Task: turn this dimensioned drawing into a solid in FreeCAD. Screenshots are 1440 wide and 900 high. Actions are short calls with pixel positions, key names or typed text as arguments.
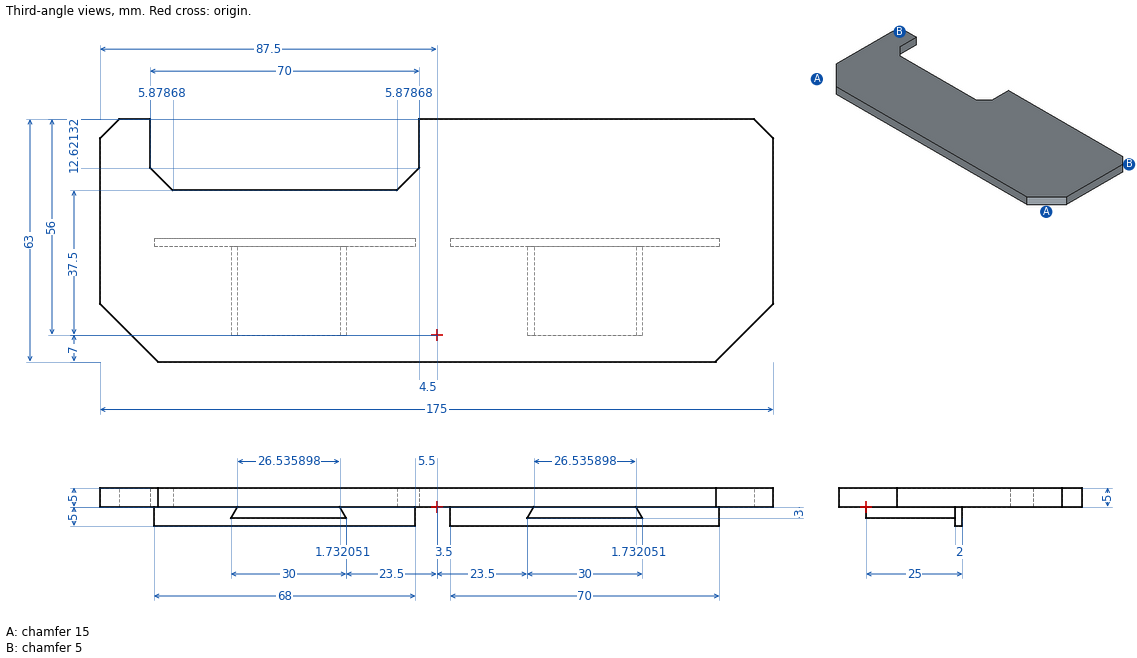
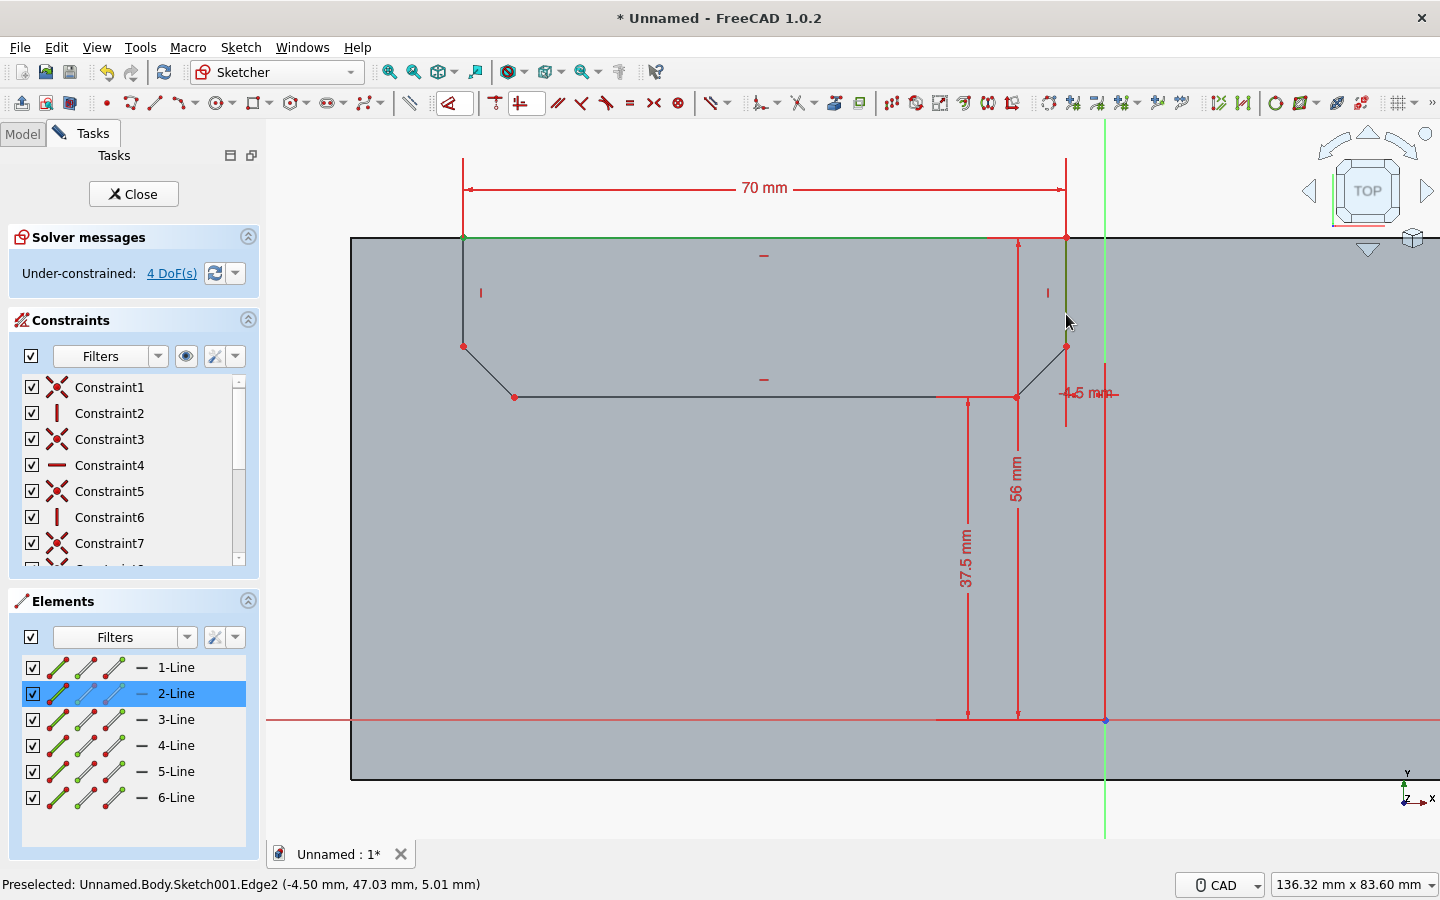
key(i)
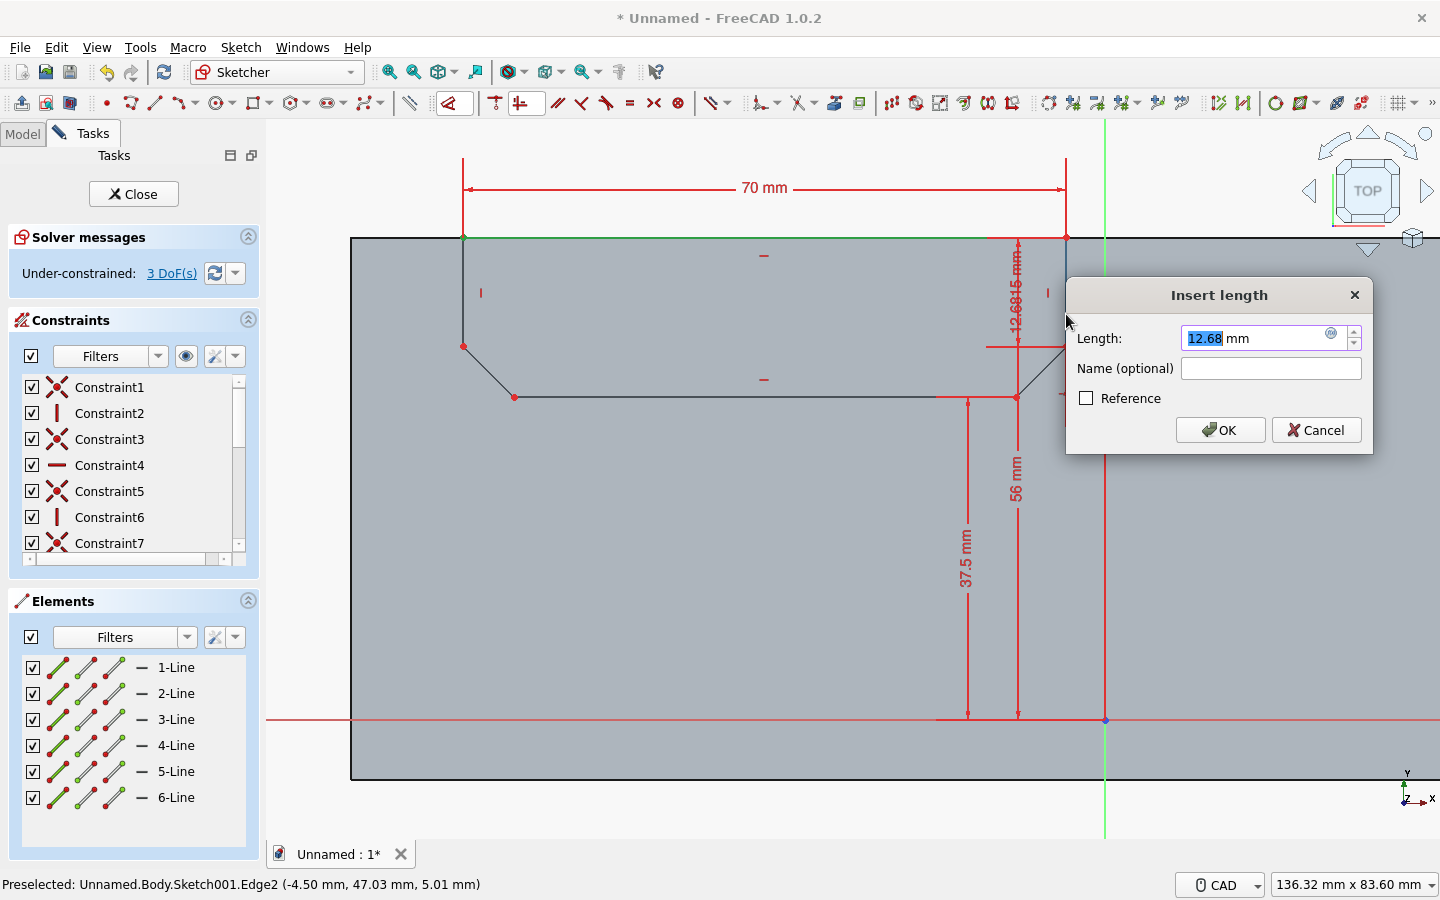
text(12.62132)
key(Return)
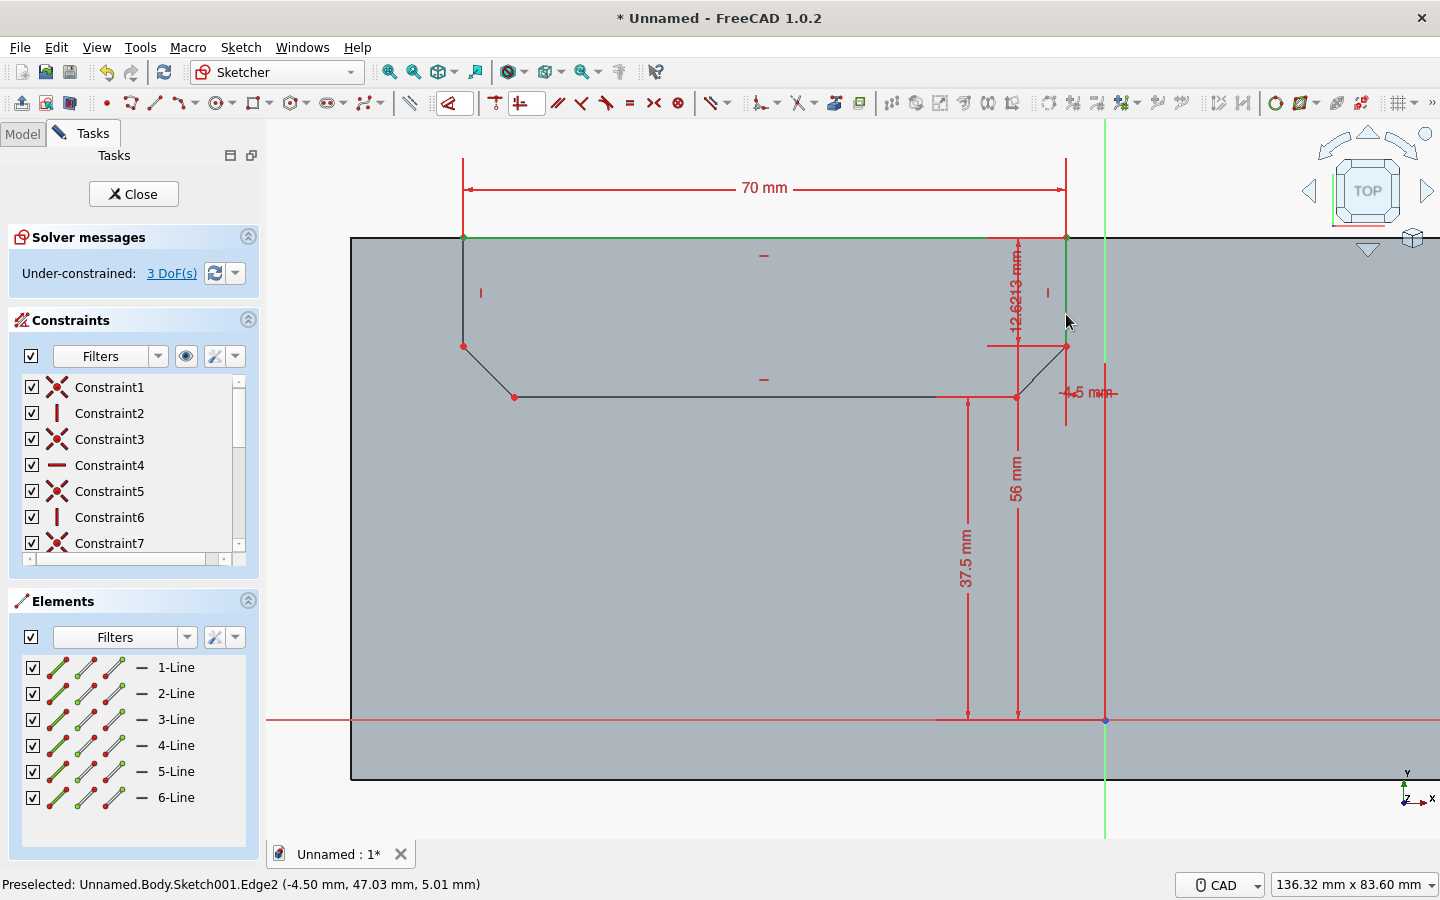
click(463, 271)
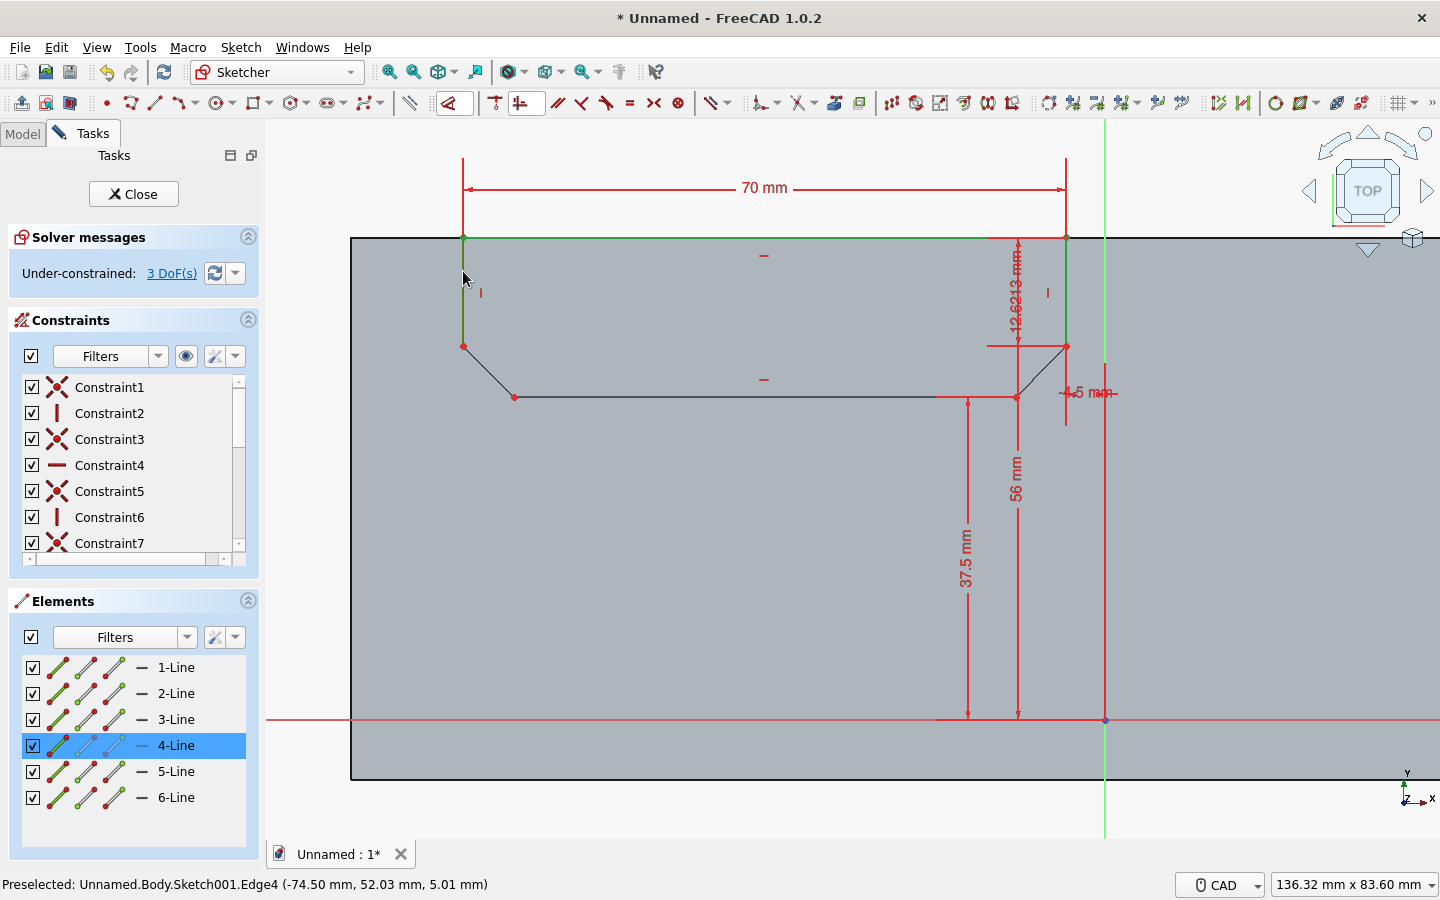
click(468, 104)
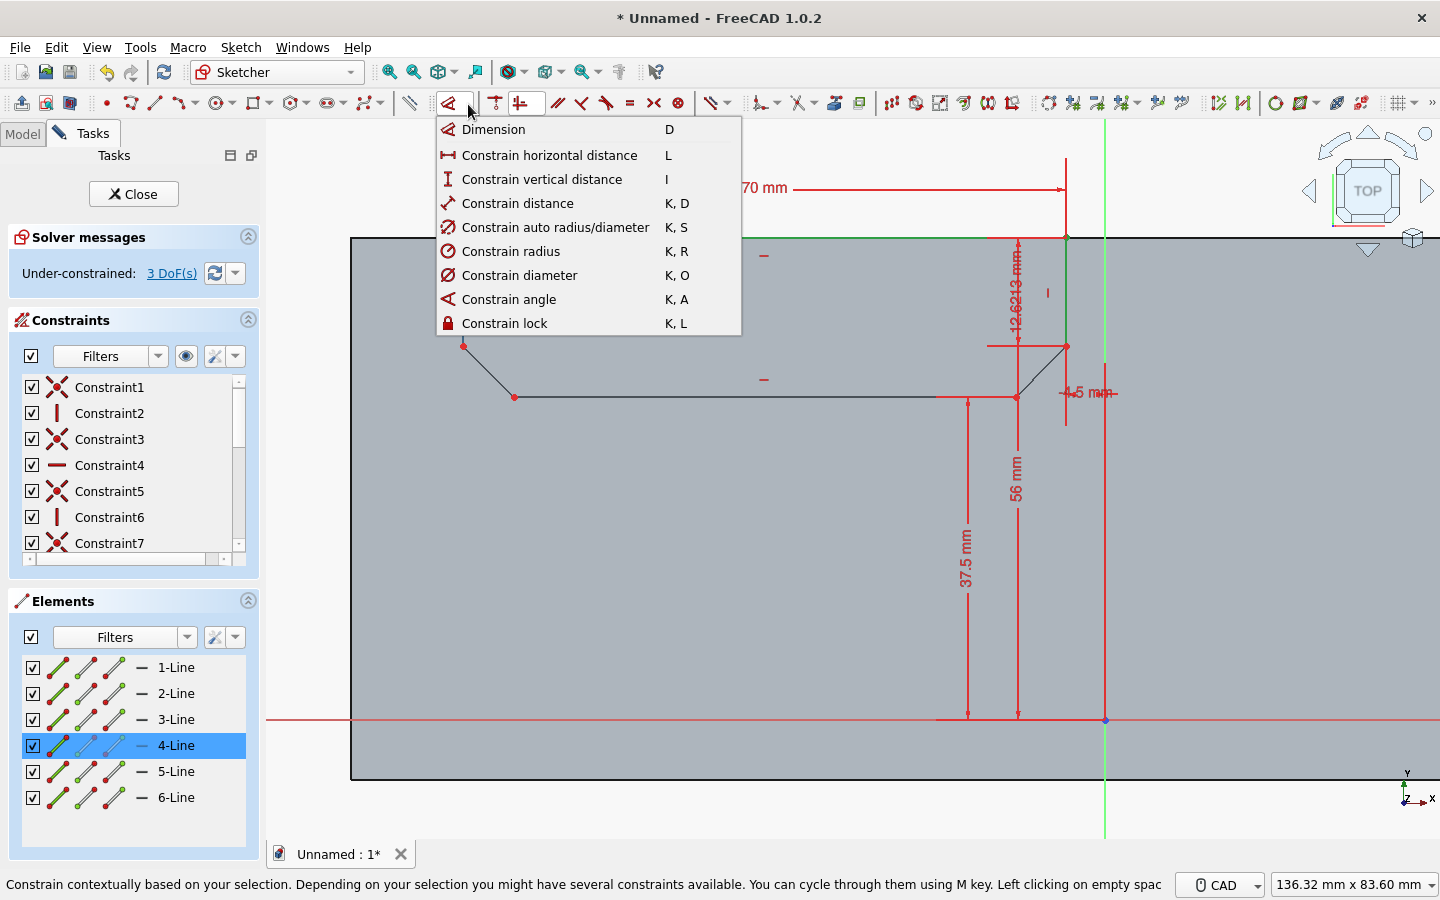
click(589, 179)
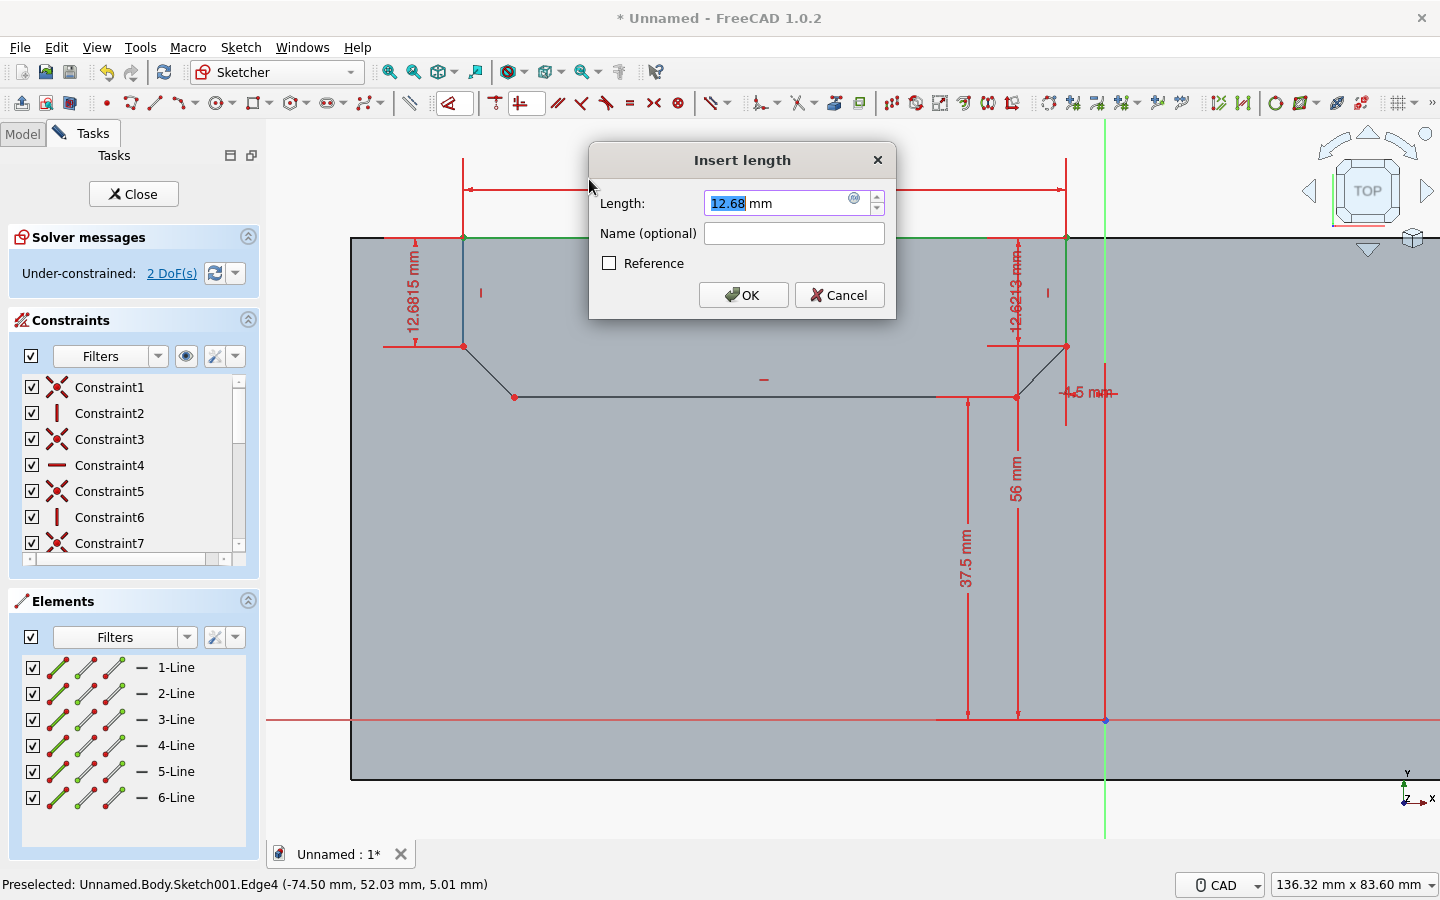
text(12.62132)
key(Return)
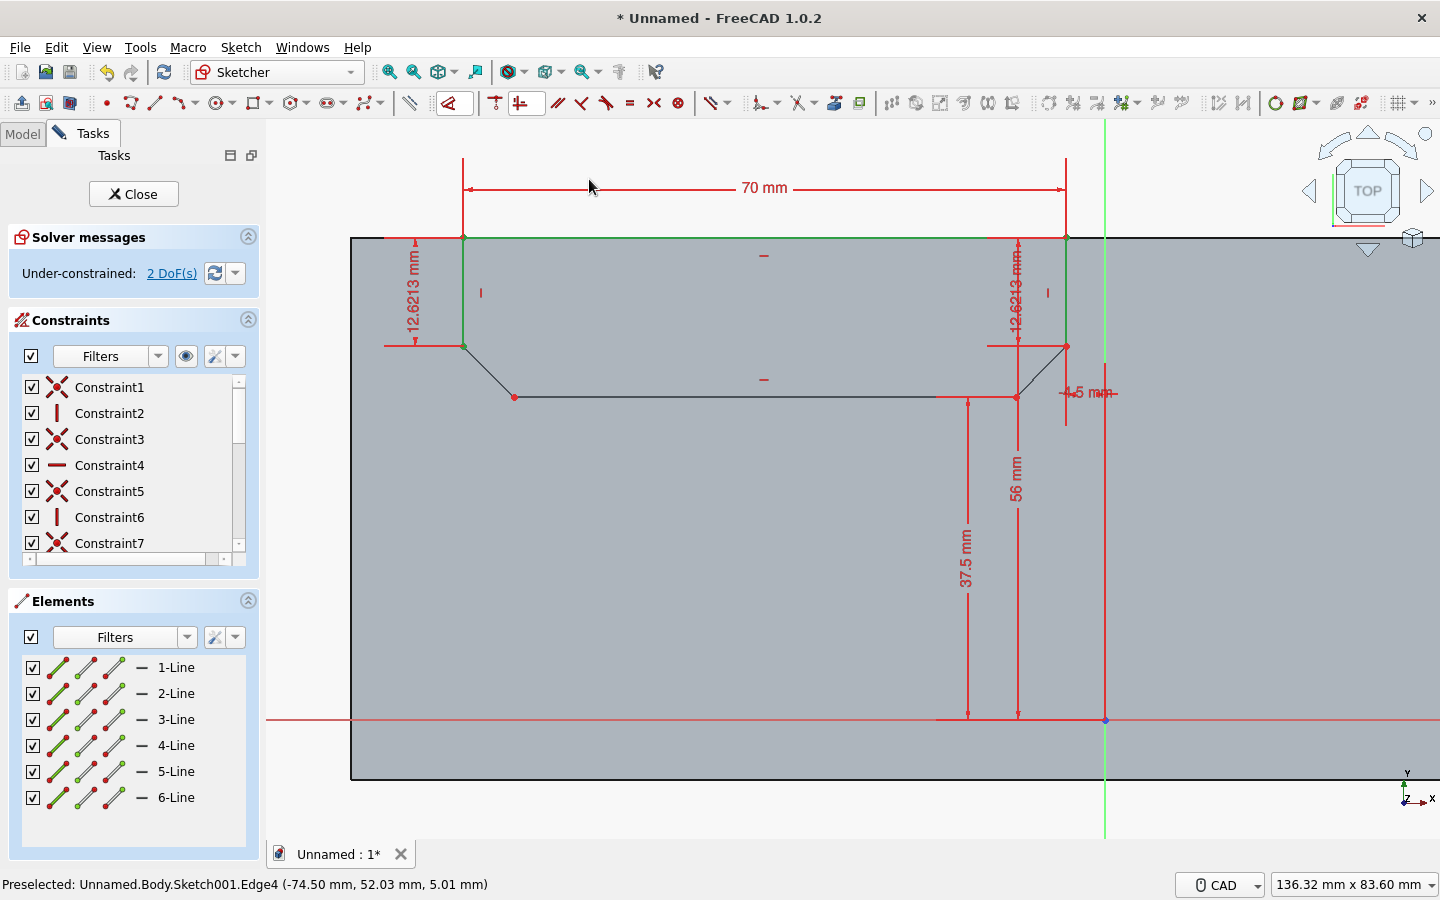
click(1031, 382)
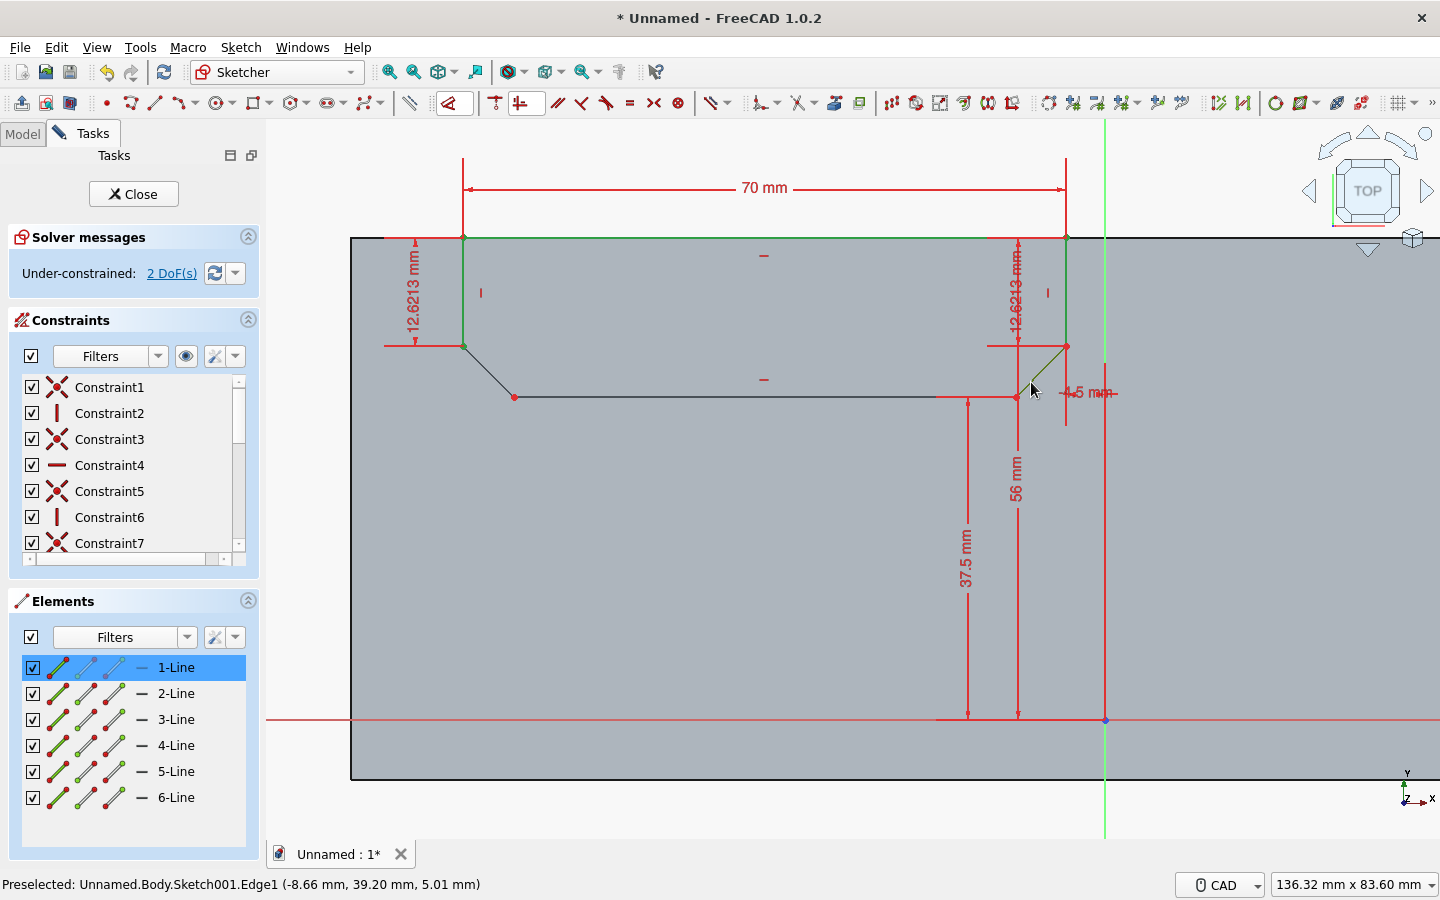
click(468, 104)